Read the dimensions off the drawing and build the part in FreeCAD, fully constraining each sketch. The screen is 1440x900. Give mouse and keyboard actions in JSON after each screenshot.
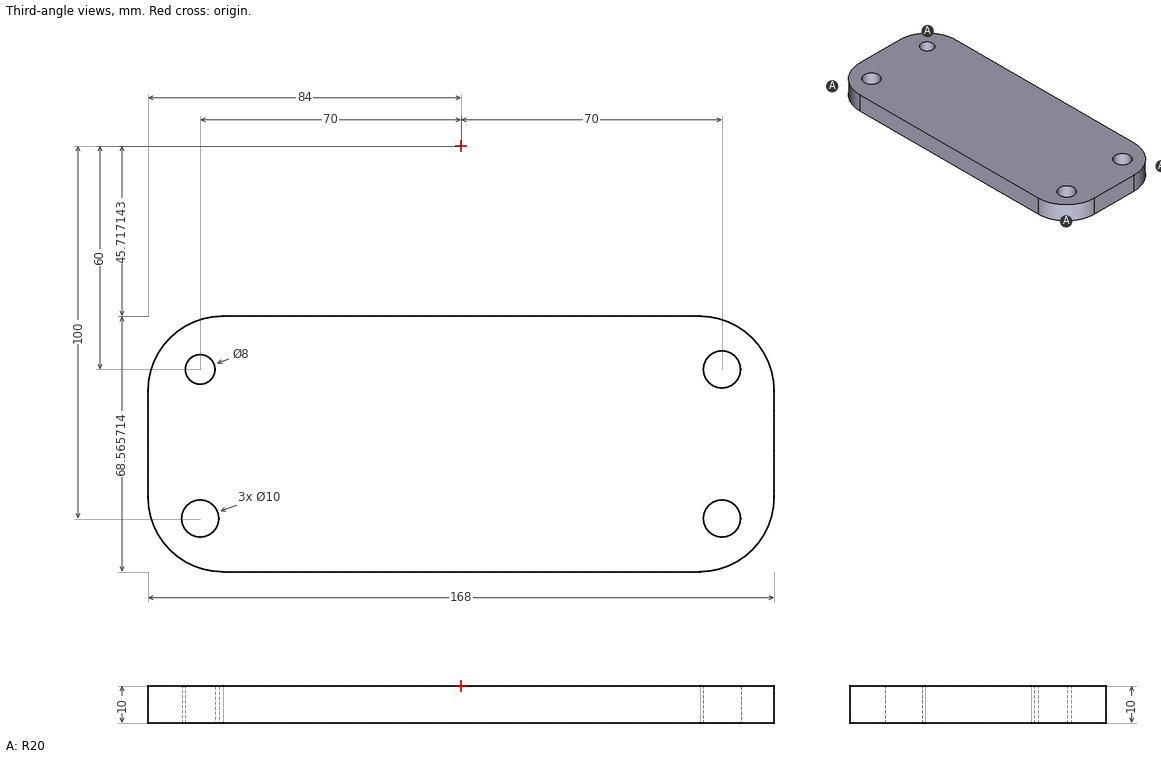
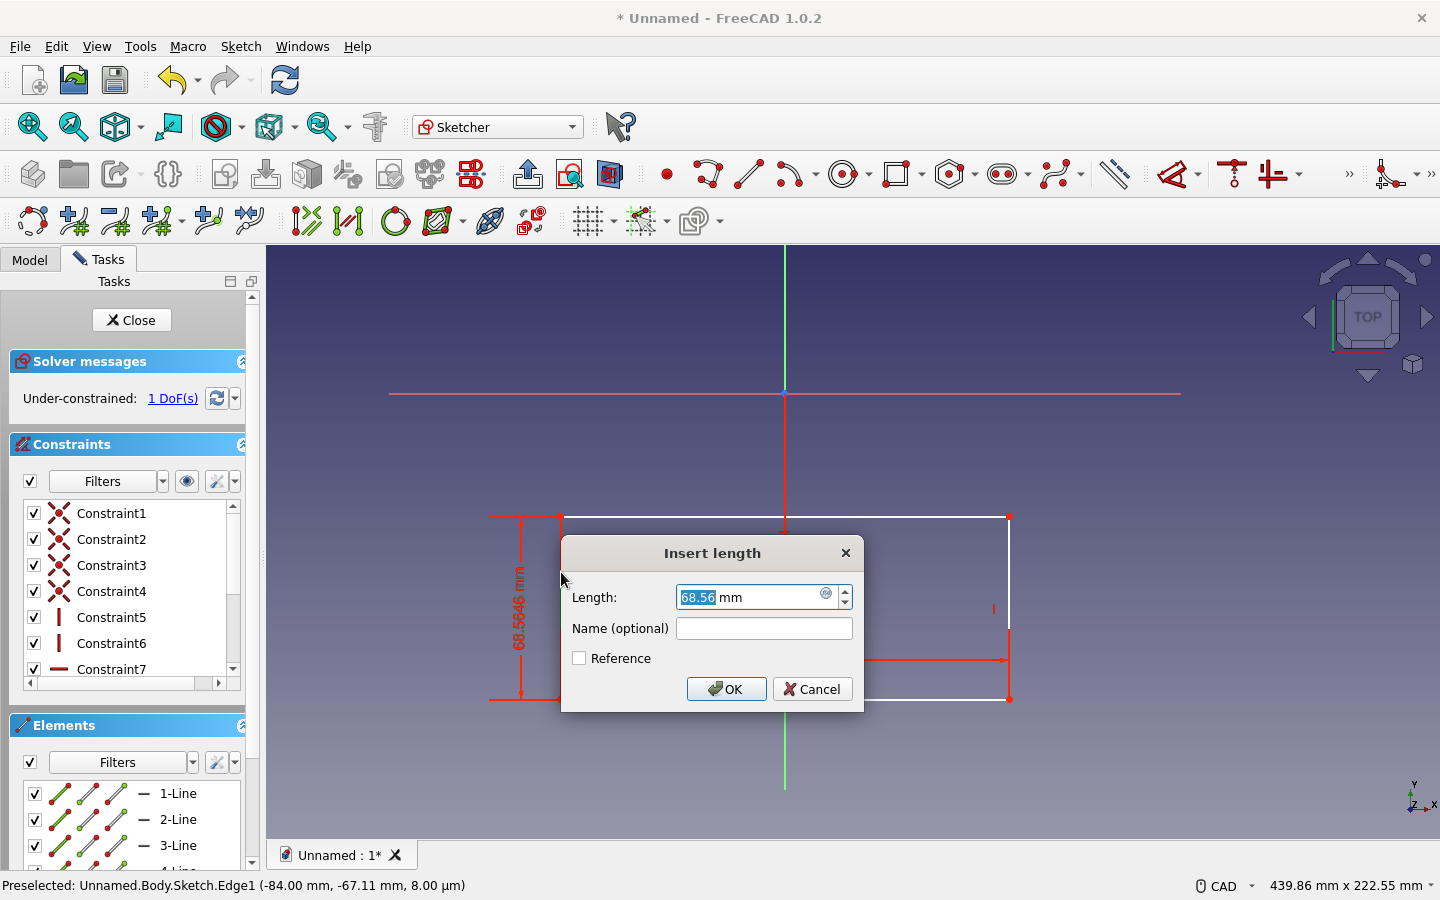
{"action": "type", "text": "68.565714"}
{"action": "key", "text": "Return"}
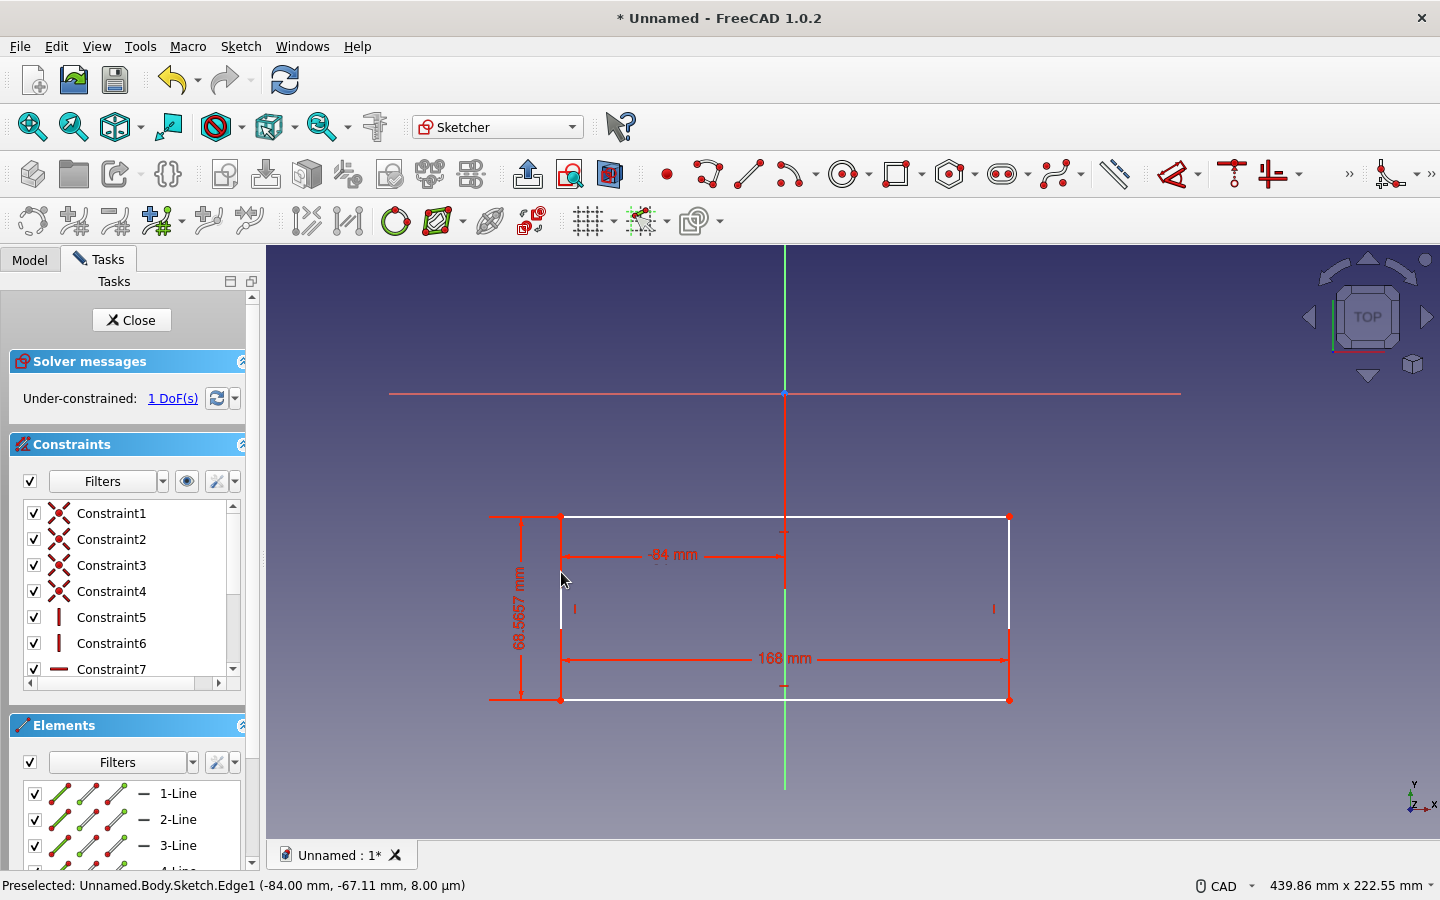
{"action": "left_click", "coordinate": [561, 517]}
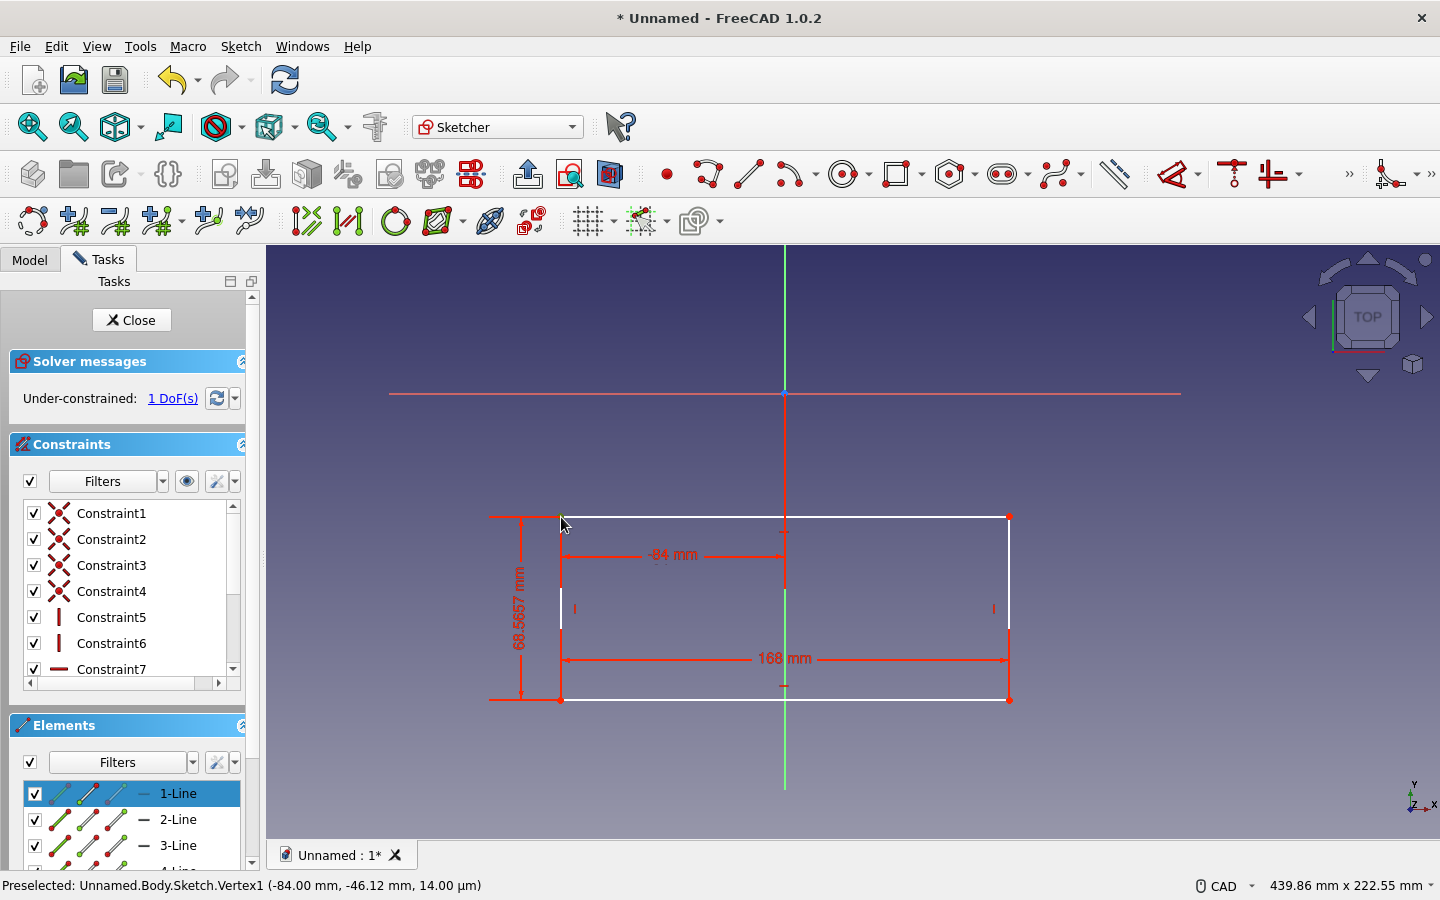
{"action": "left_click", "coordinate": [1198, 174]}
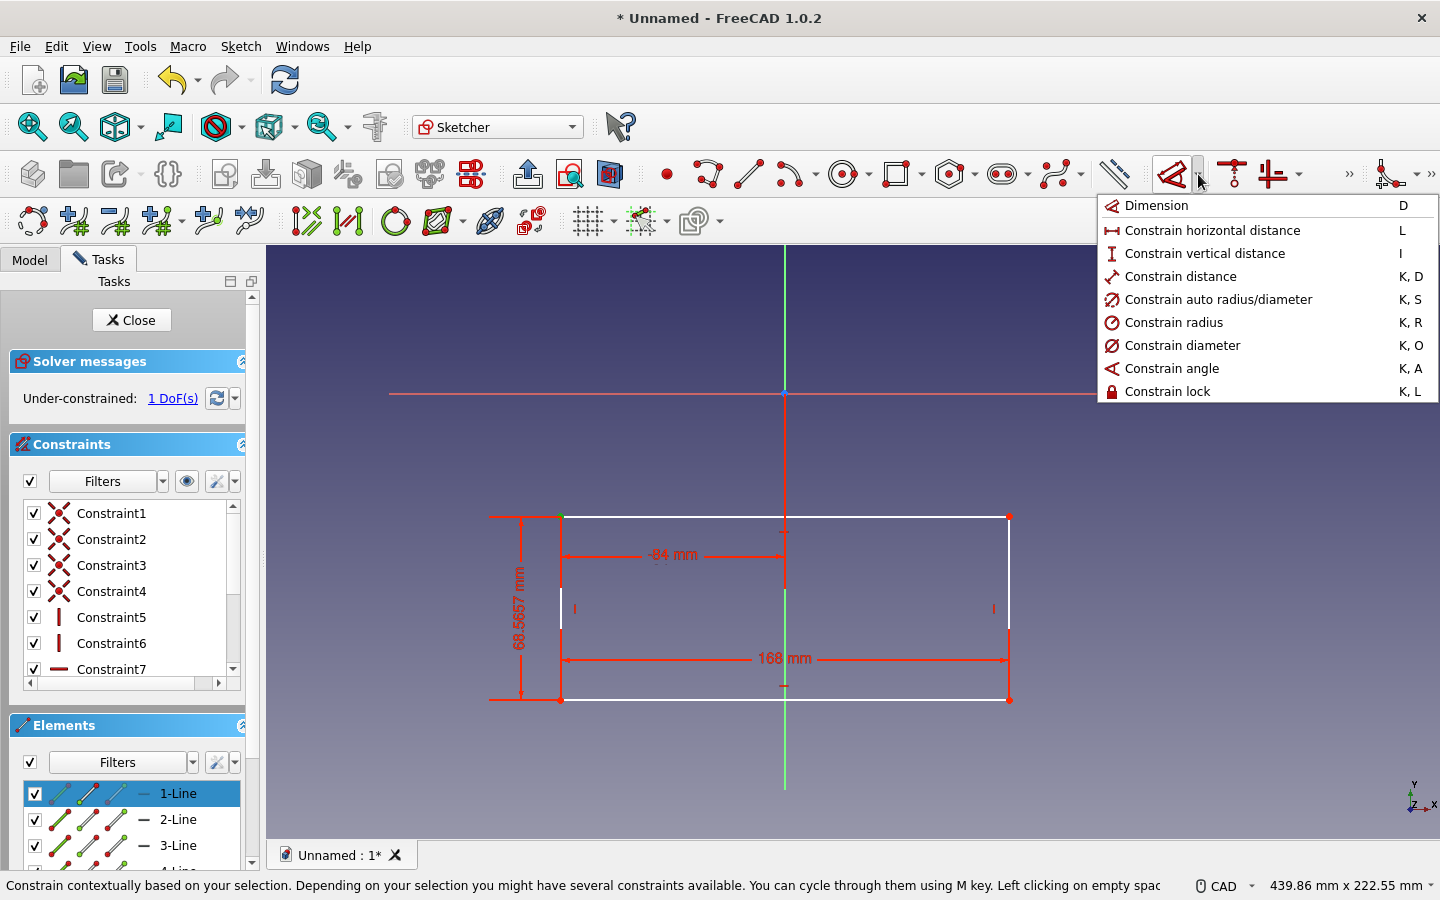
{"action": "left_click", "coordinate": [1268, 254]}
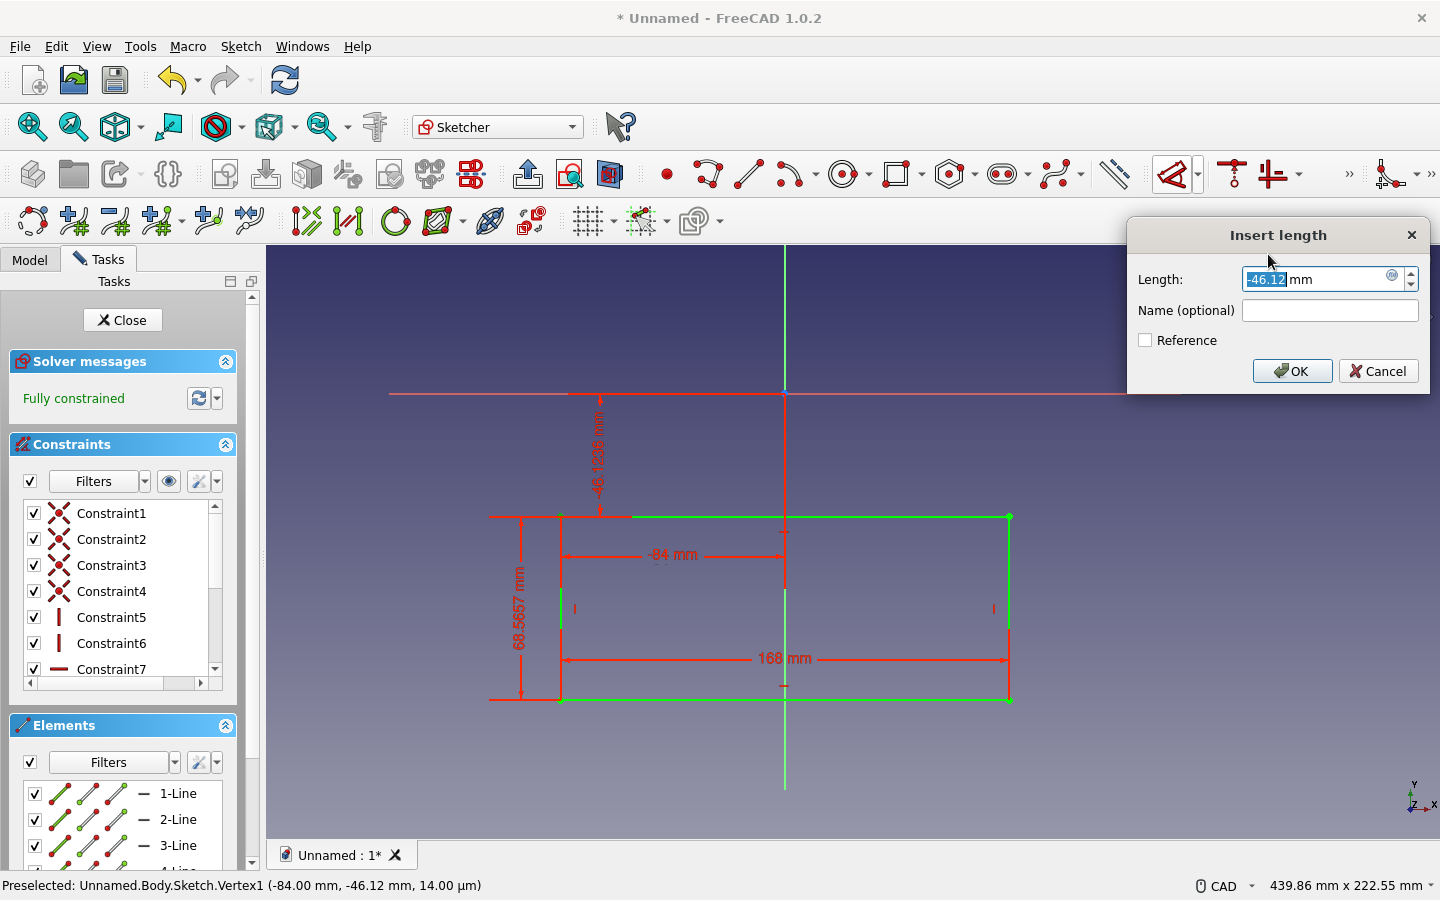
{"action": "type", "text": "-45.717143"}
{"action": "key", "text": "Return"}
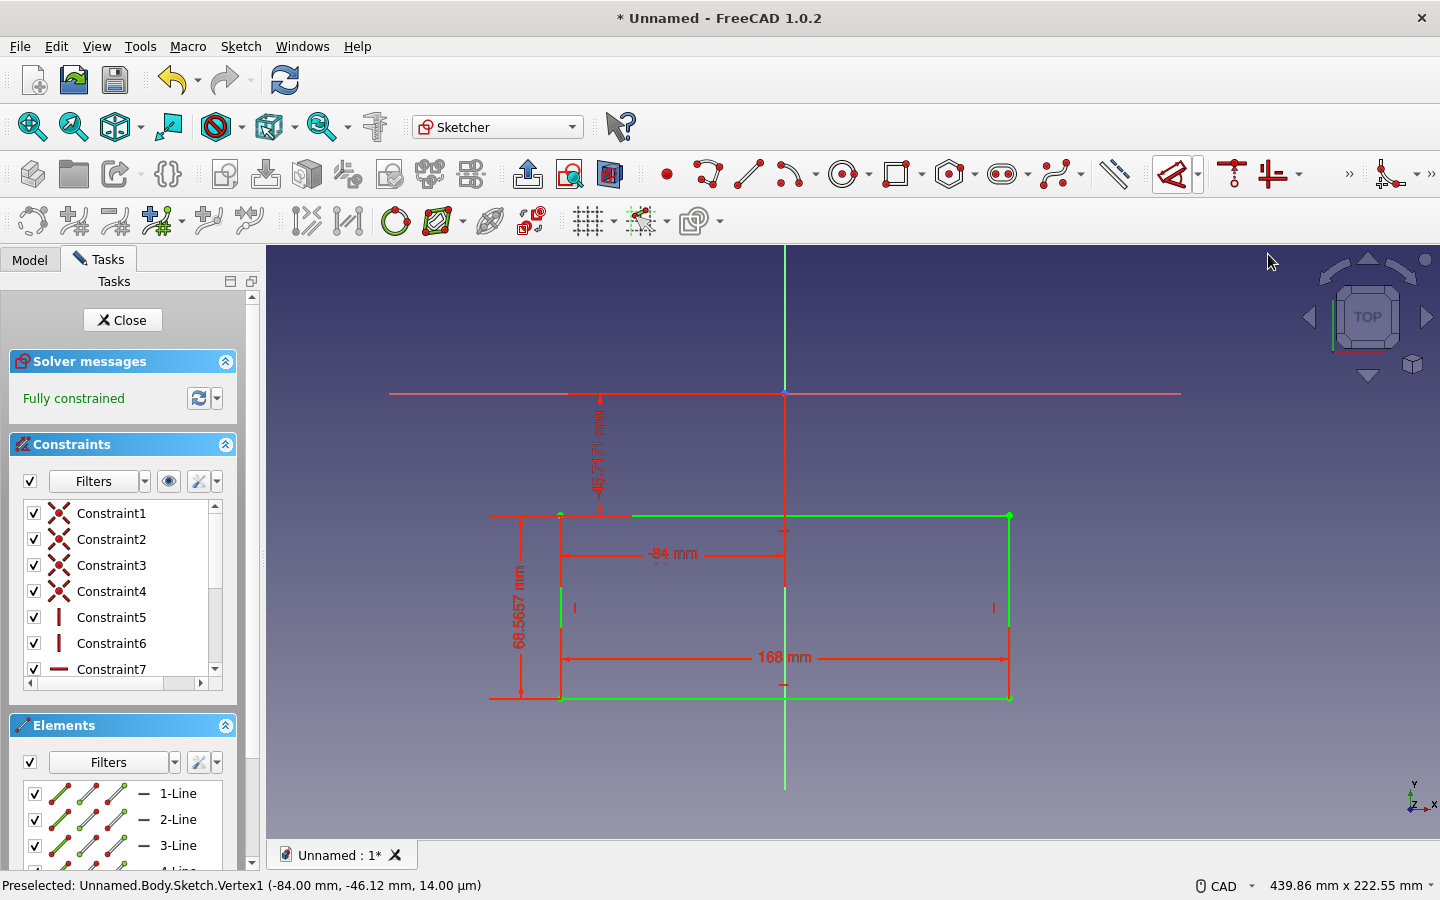
{"action": "left_click", "coordinate": [123, 320]}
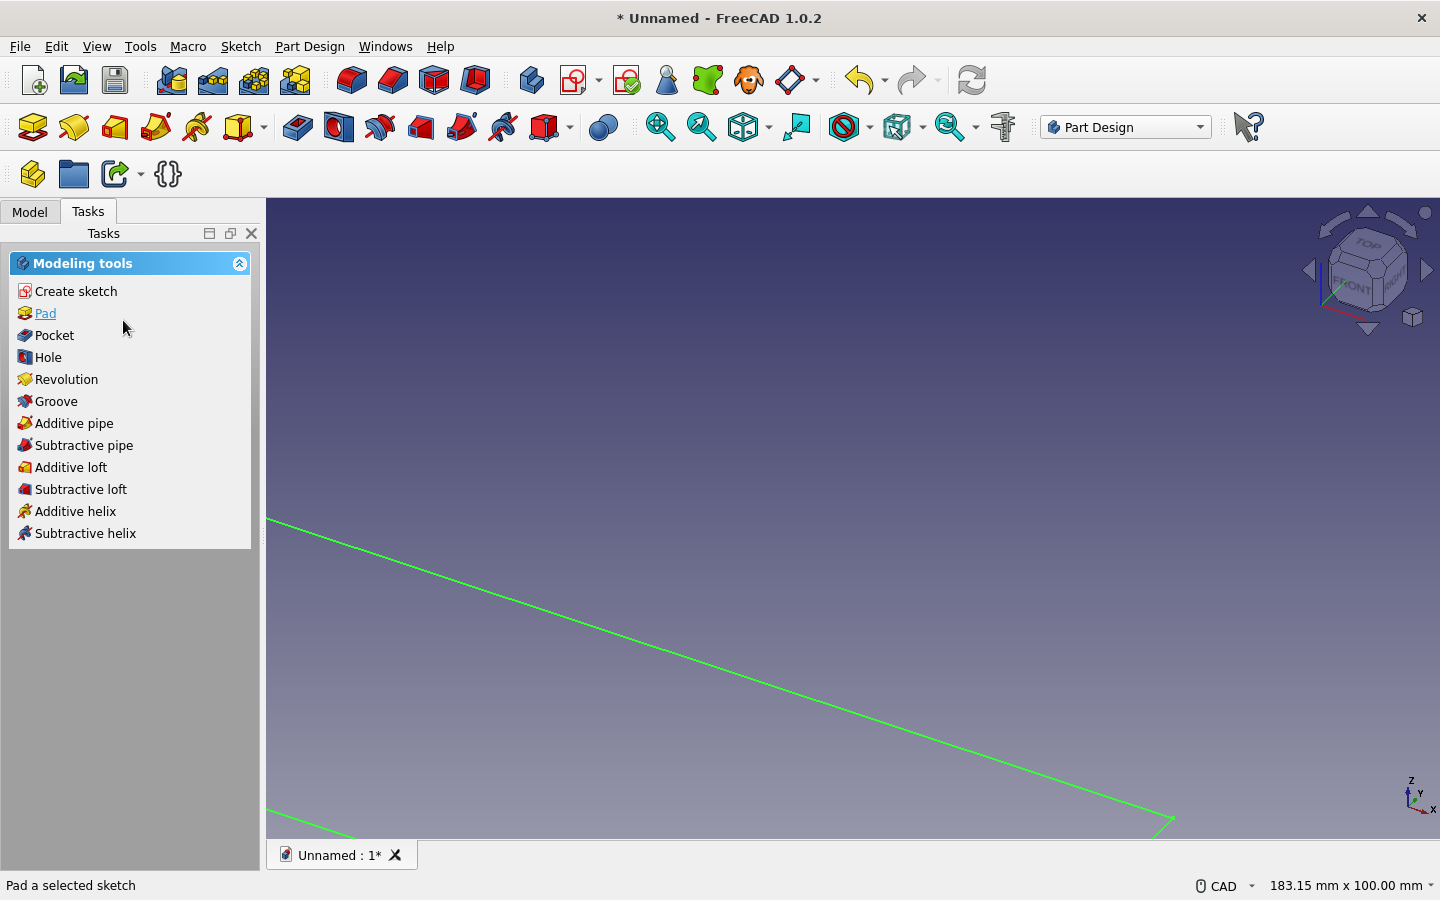
{"action": "left_click", "coordinate": [33, 128]}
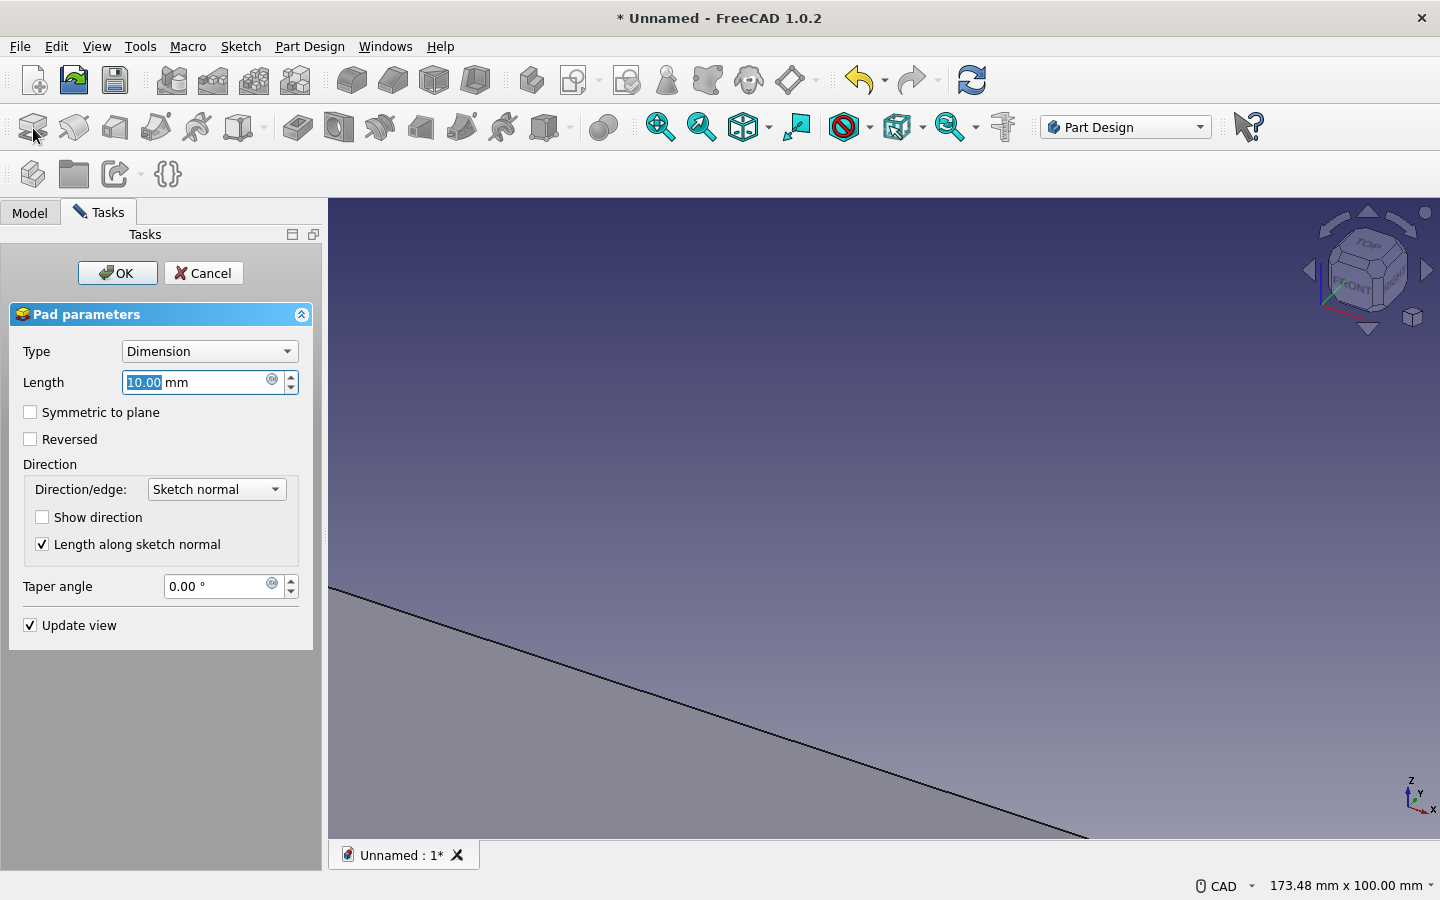
{"action": "type", "text": "10"}
{"action": "key", "text": "Tab"}